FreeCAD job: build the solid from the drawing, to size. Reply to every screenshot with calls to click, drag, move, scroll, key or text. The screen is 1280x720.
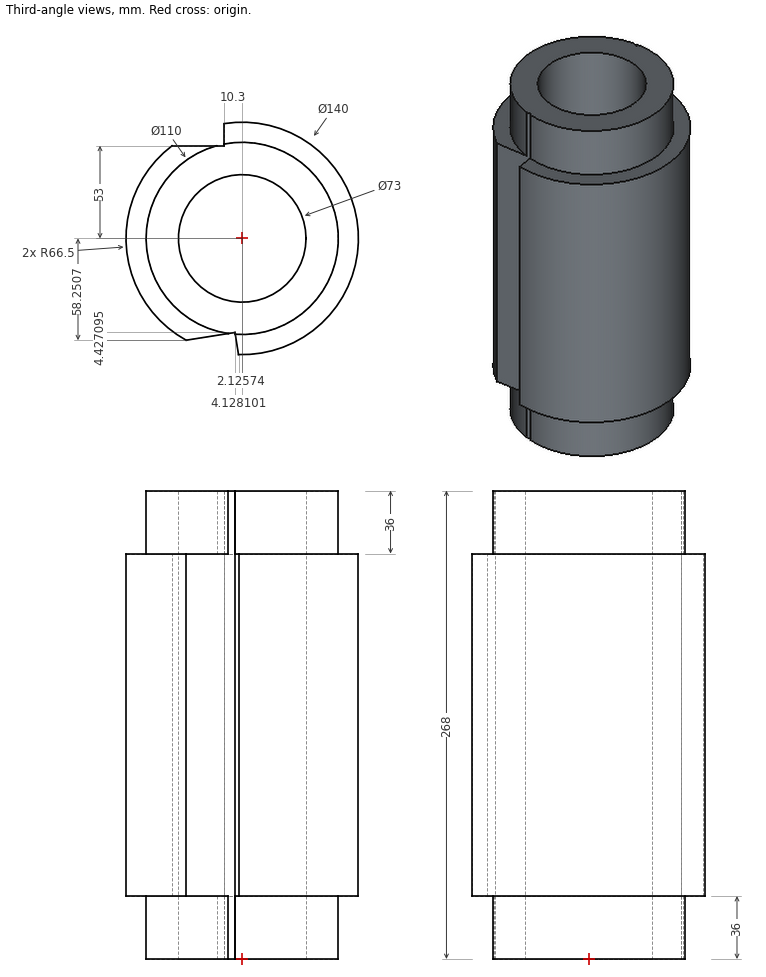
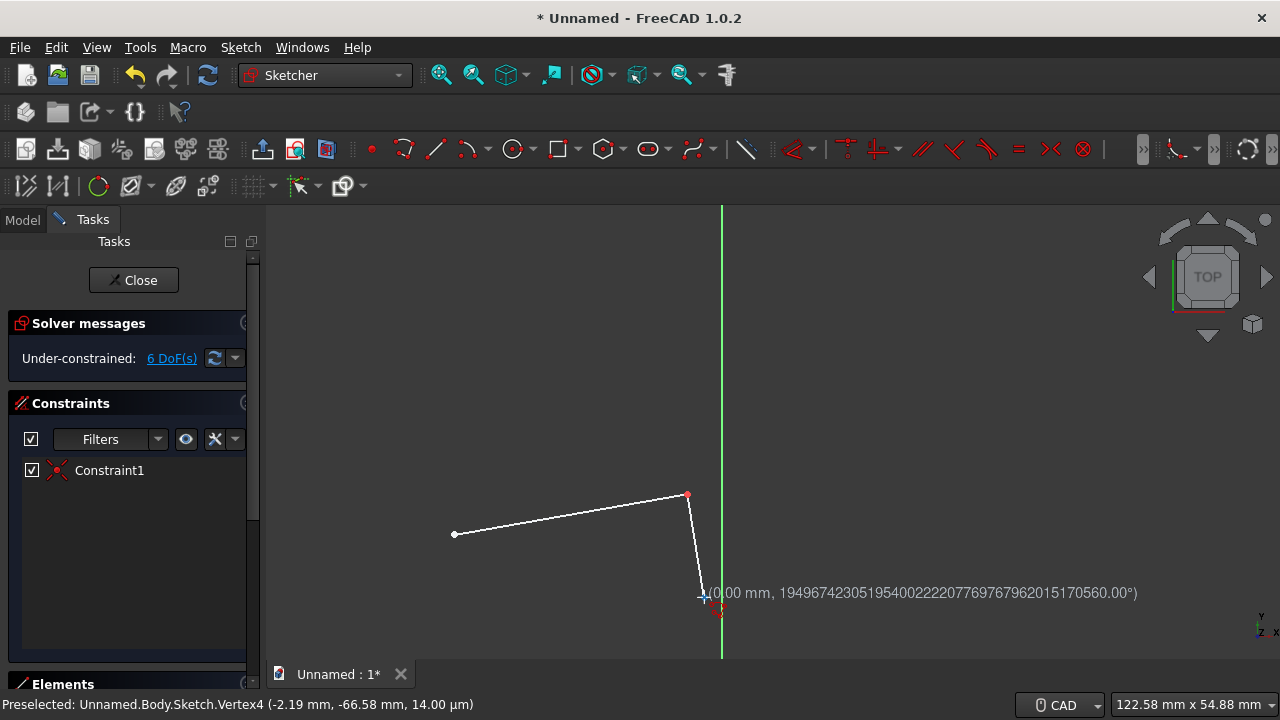
scroll(699, 557, down, 7)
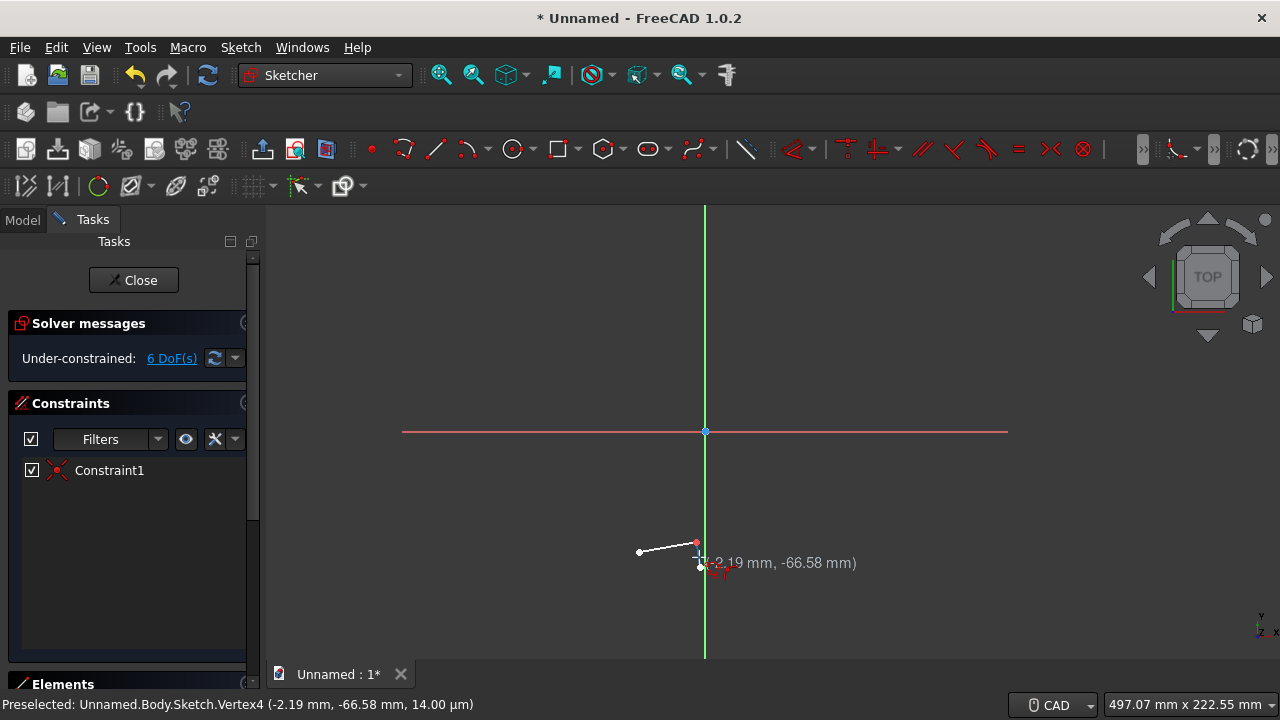
click(684, 298)
click(684, 324)
click(623, 324)
right_click(623, 324)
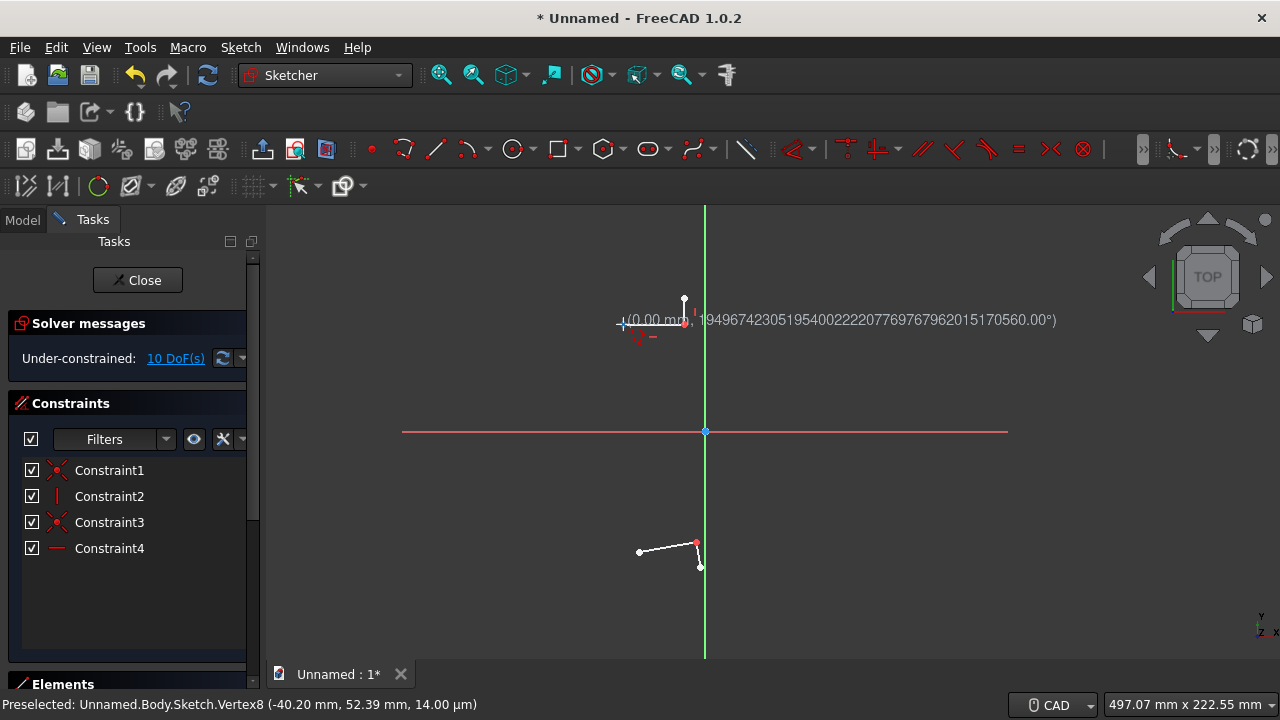
click(490, 150)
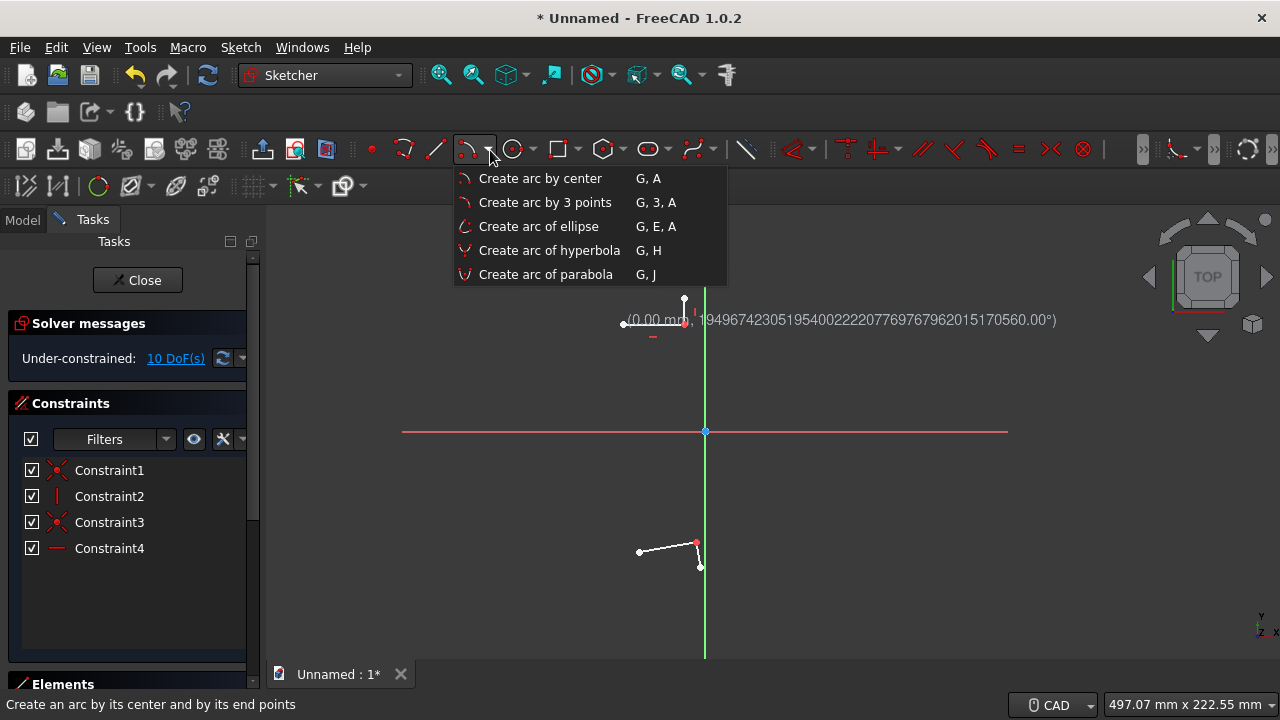
click(590, 202)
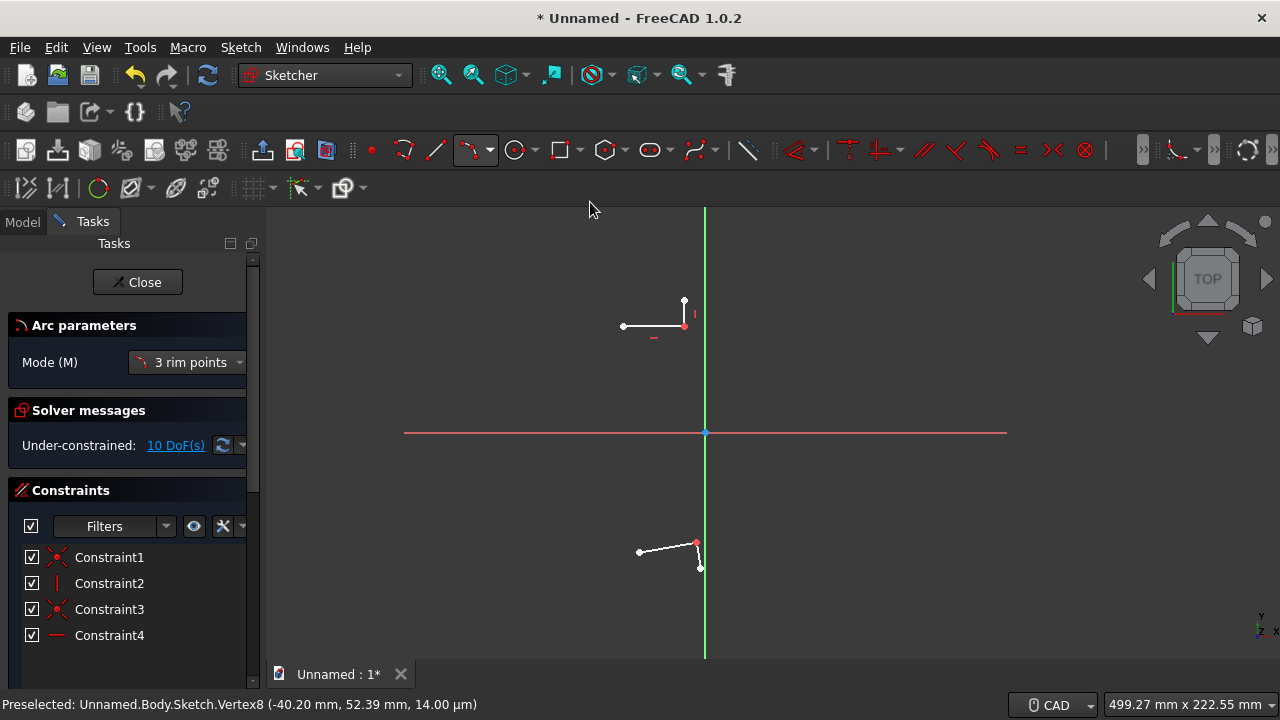
scroll(701, 568, up, 7)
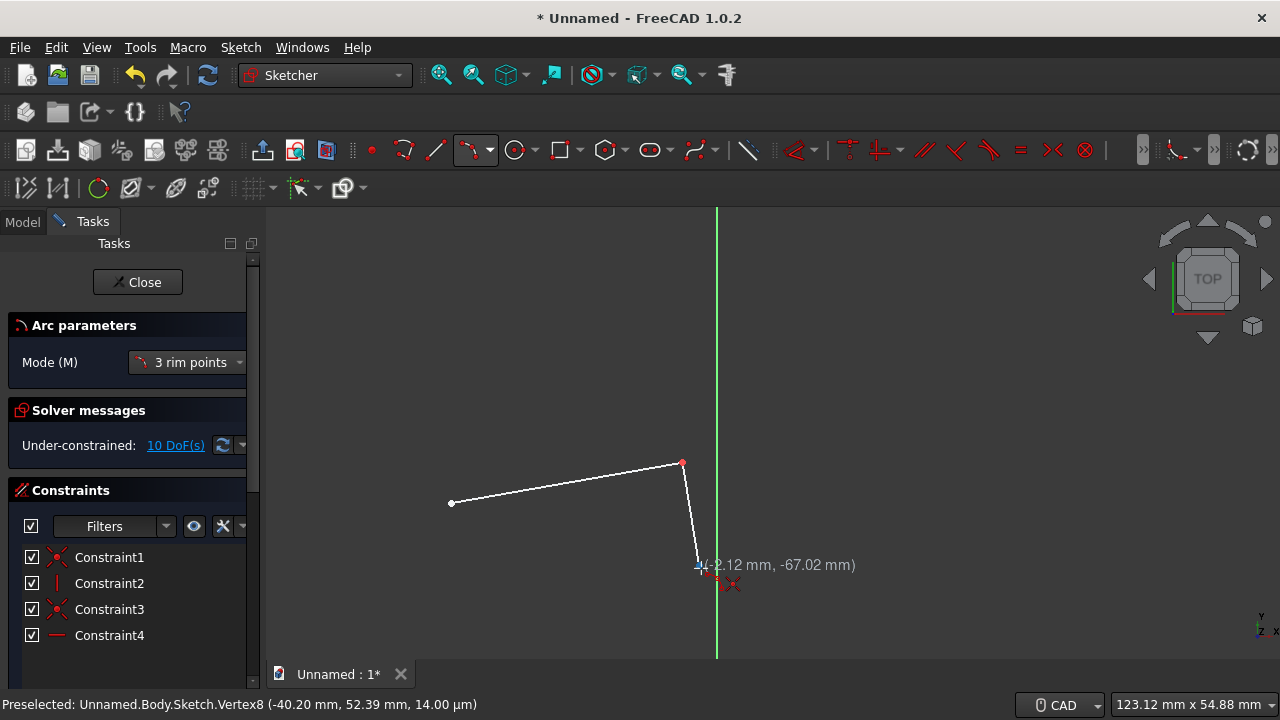
click(699, 566)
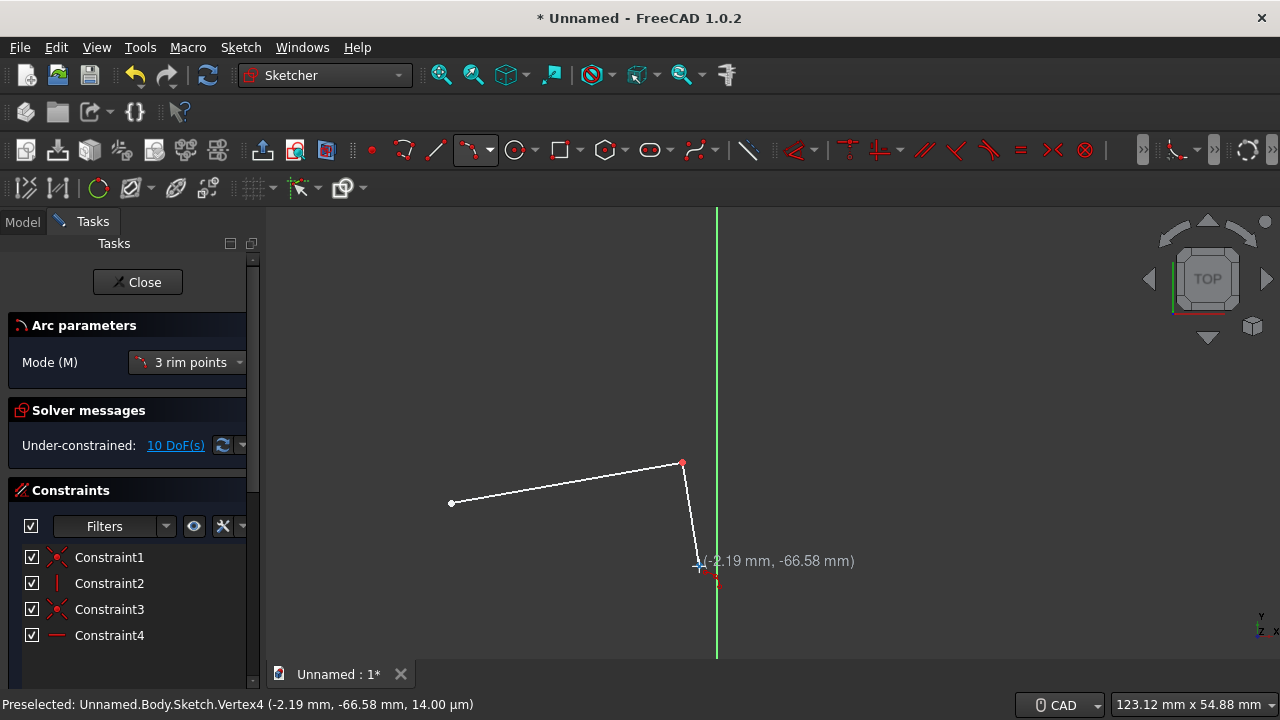
scroll(700, 568, down, 7)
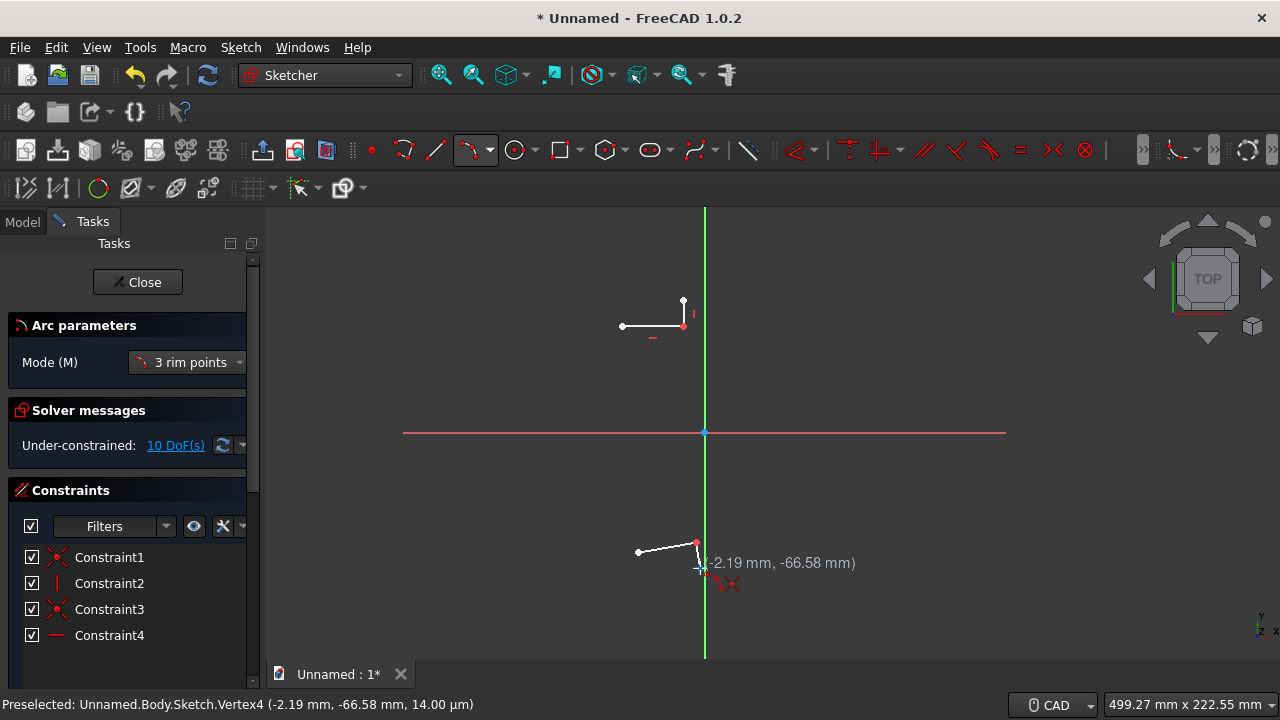
scroll(684, 299, up, 2)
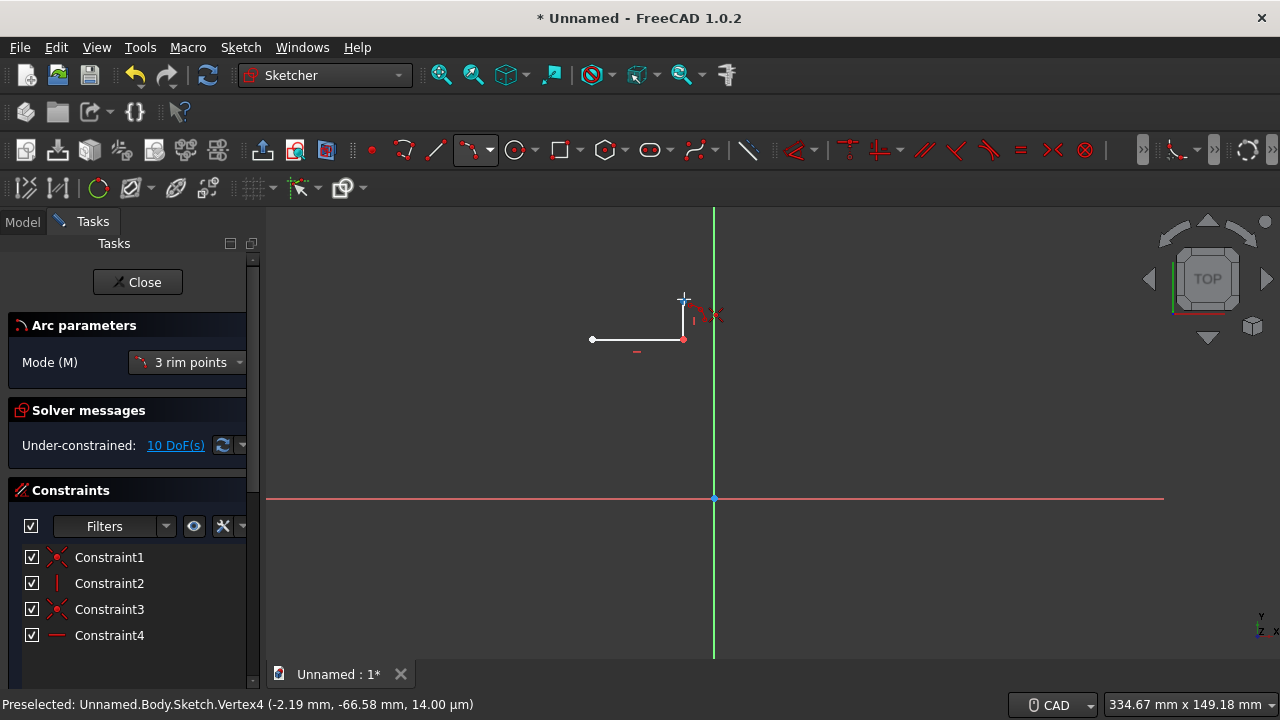
click(683, 301)
click(909, 553)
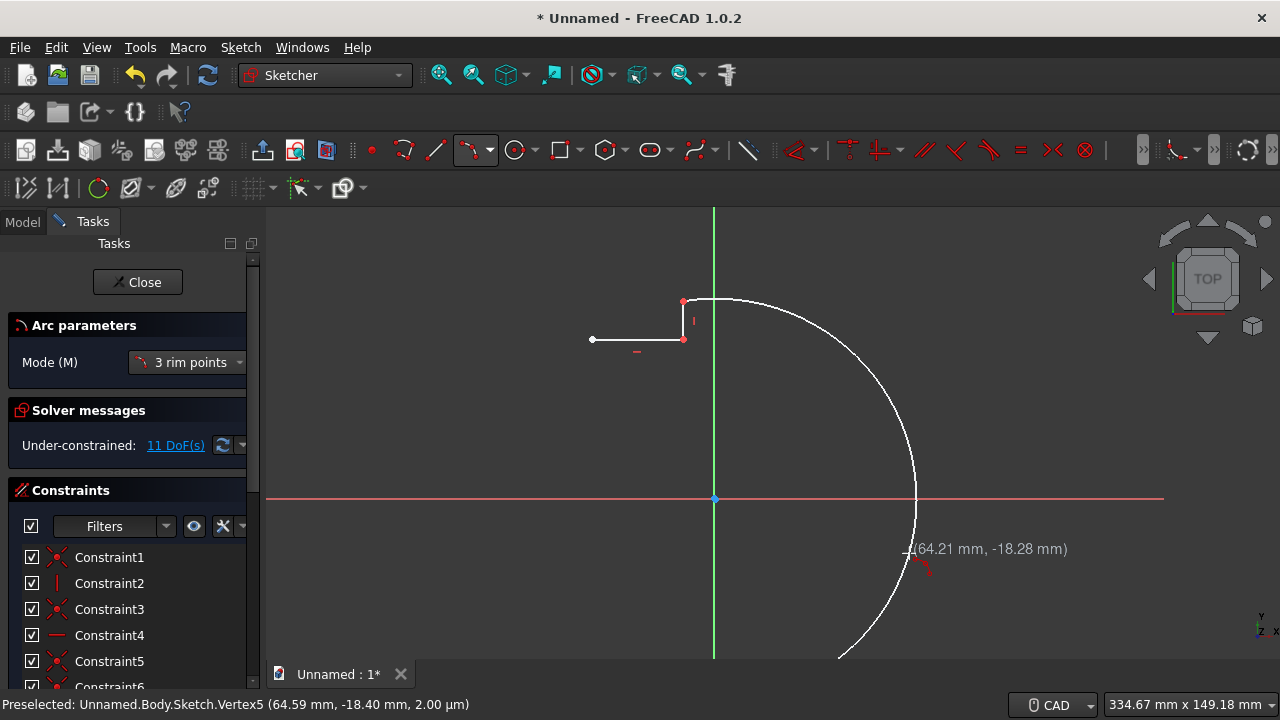
click(593, 340)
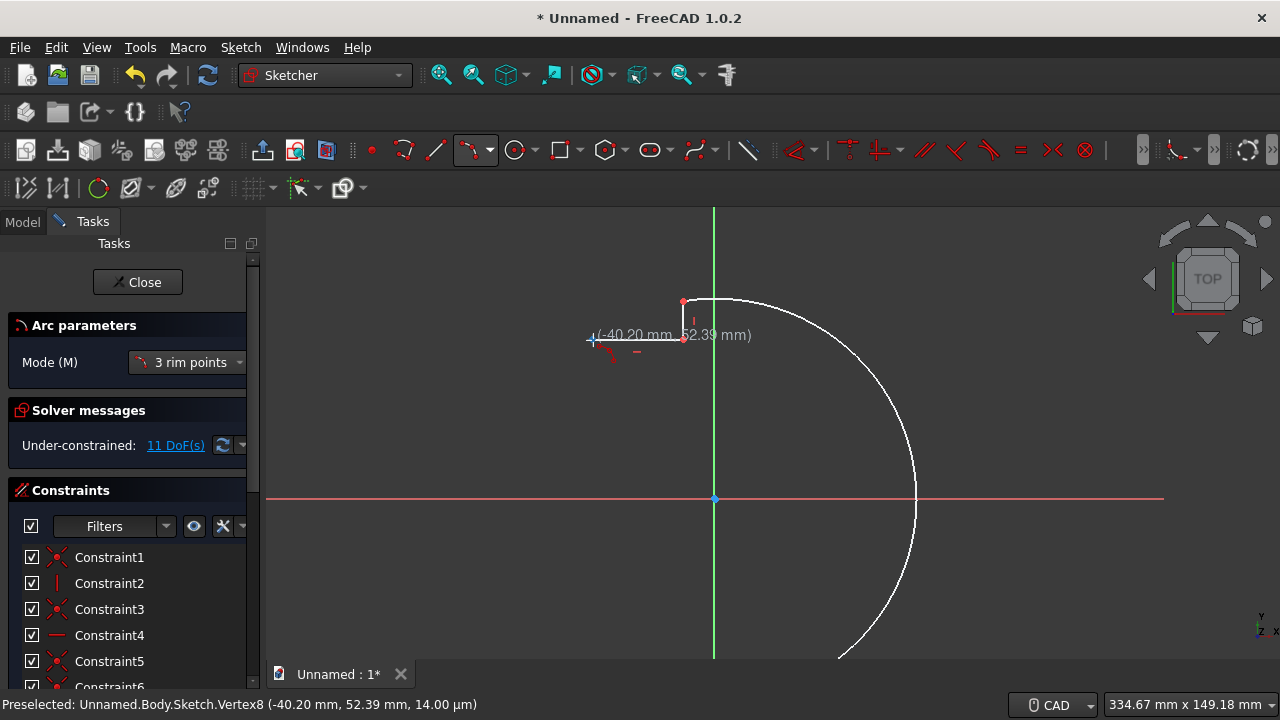
scroll(684, 297, down, 2)